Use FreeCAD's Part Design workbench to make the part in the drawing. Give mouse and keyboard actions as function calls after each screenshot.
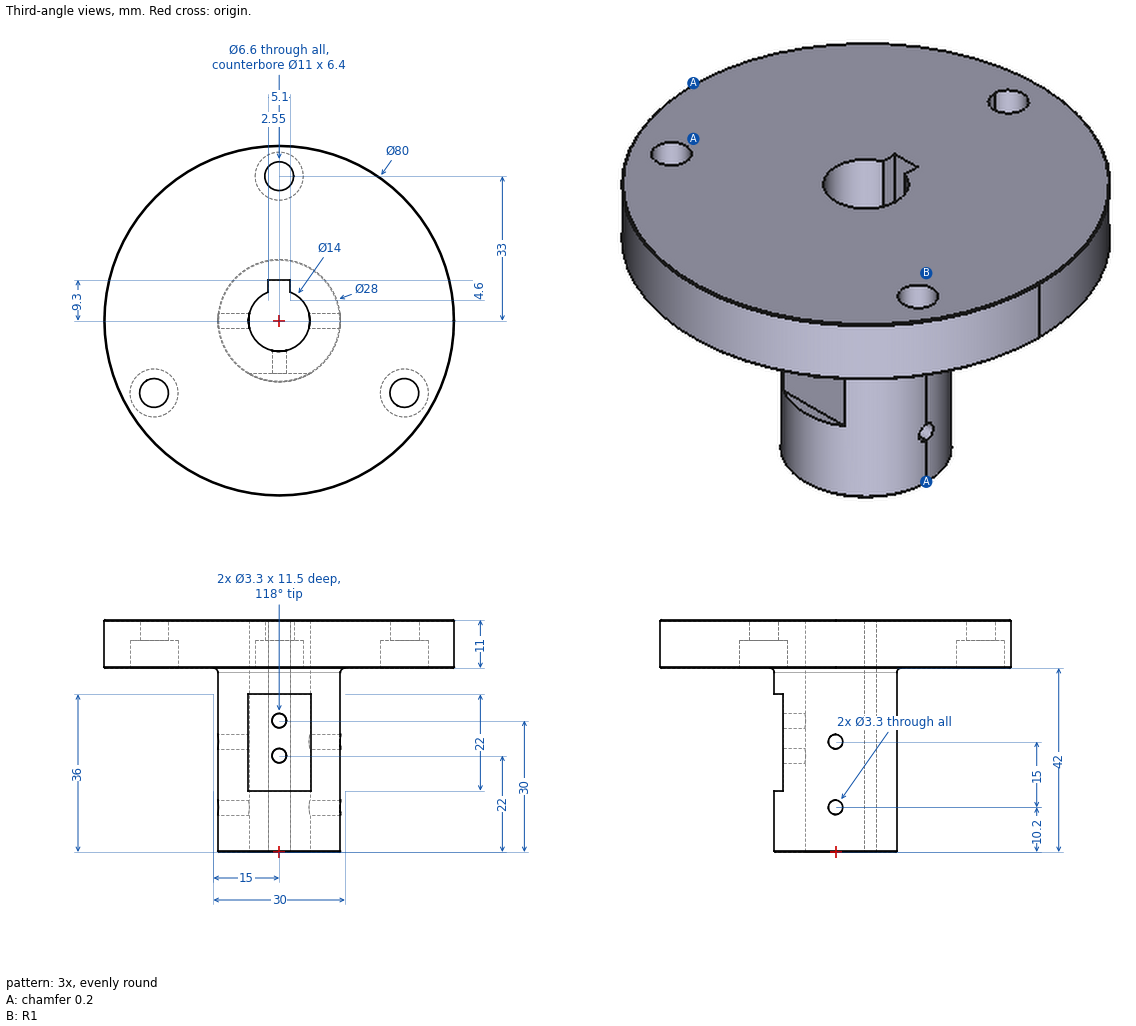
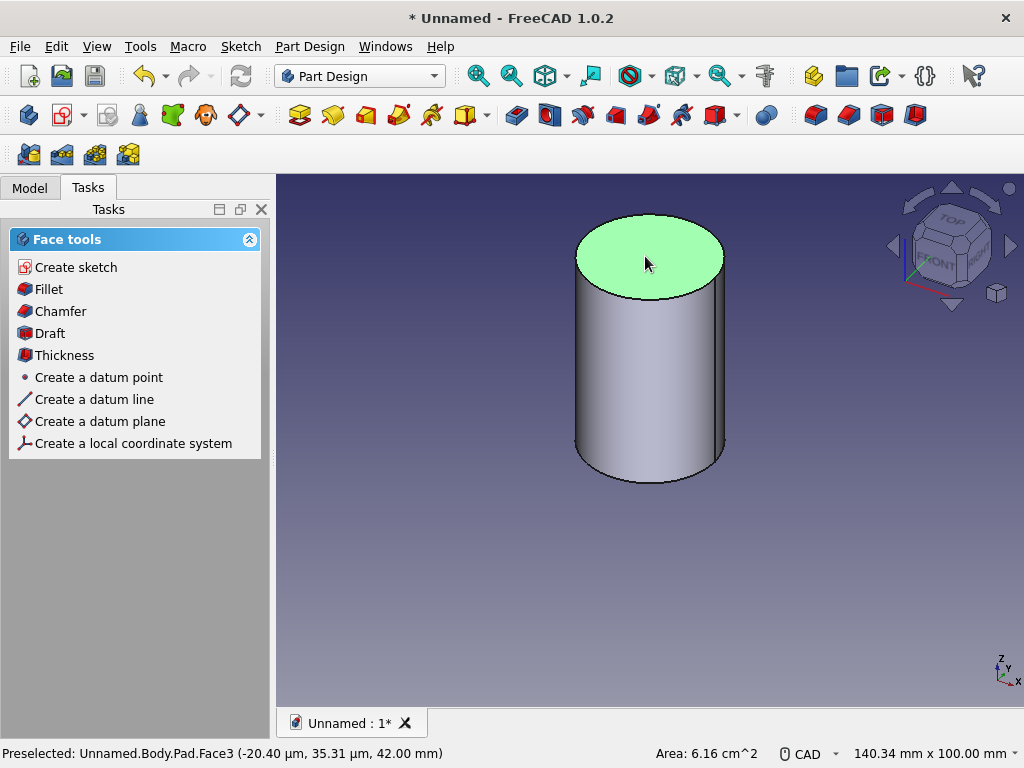
click(62, 116)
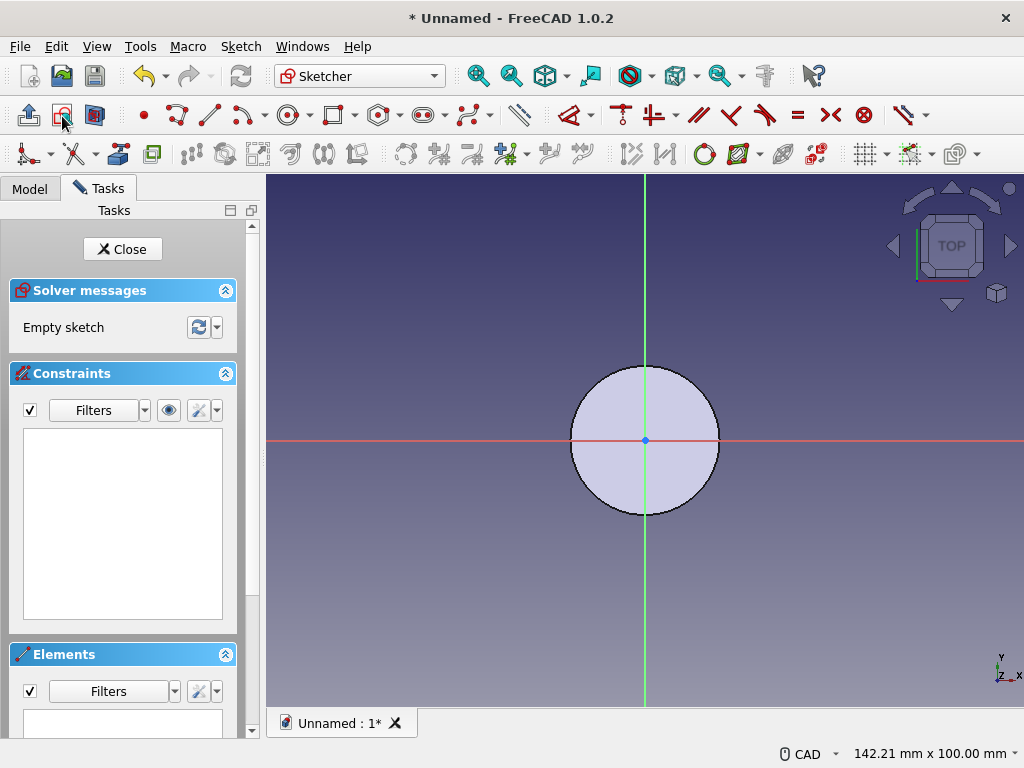
scroll(294, 440, down, 1)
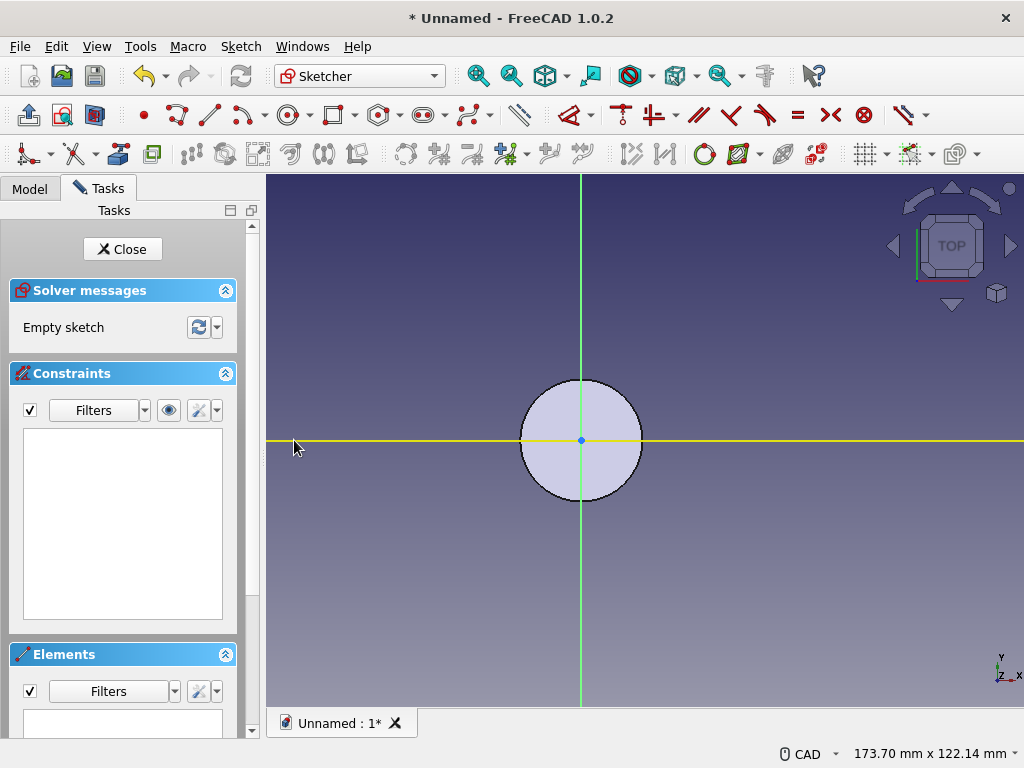
key(g)
key(c)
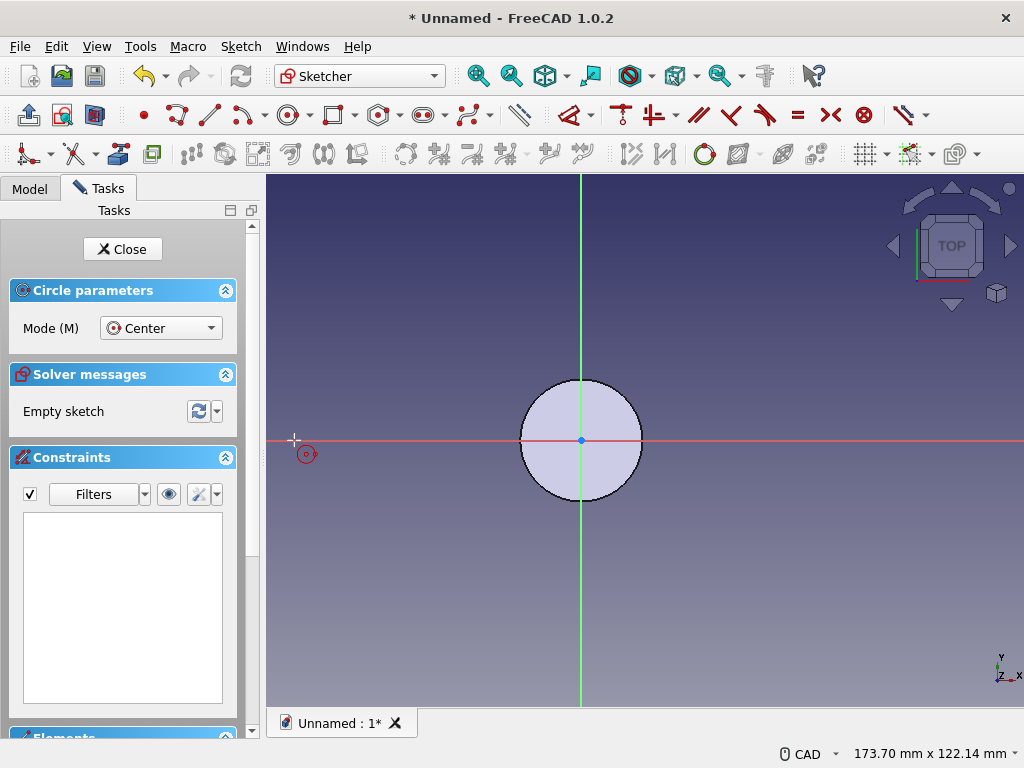
click(581, 440)
move(705, 317)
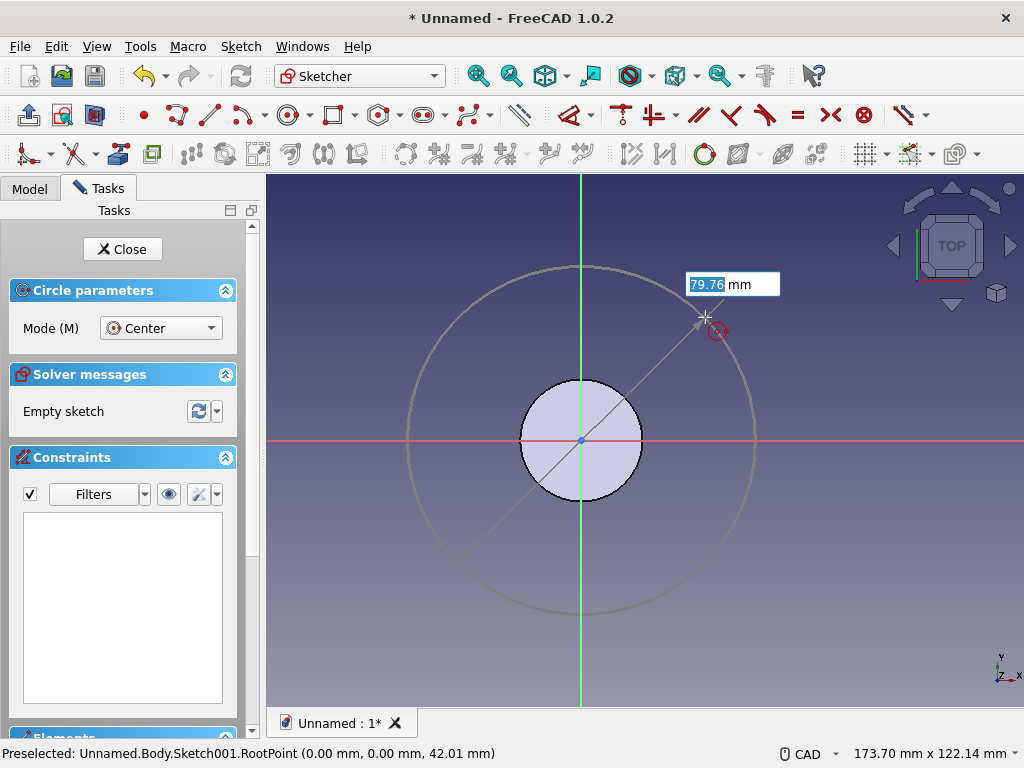
text(80)
key(Return)
key(Escape)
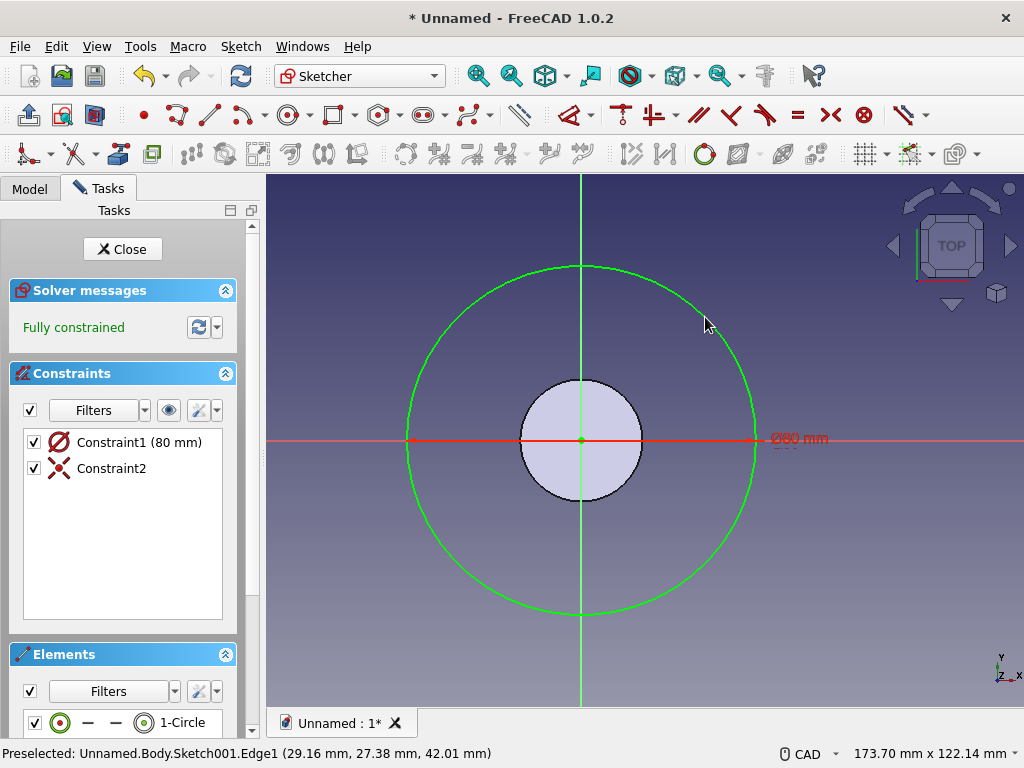
click(123, 249)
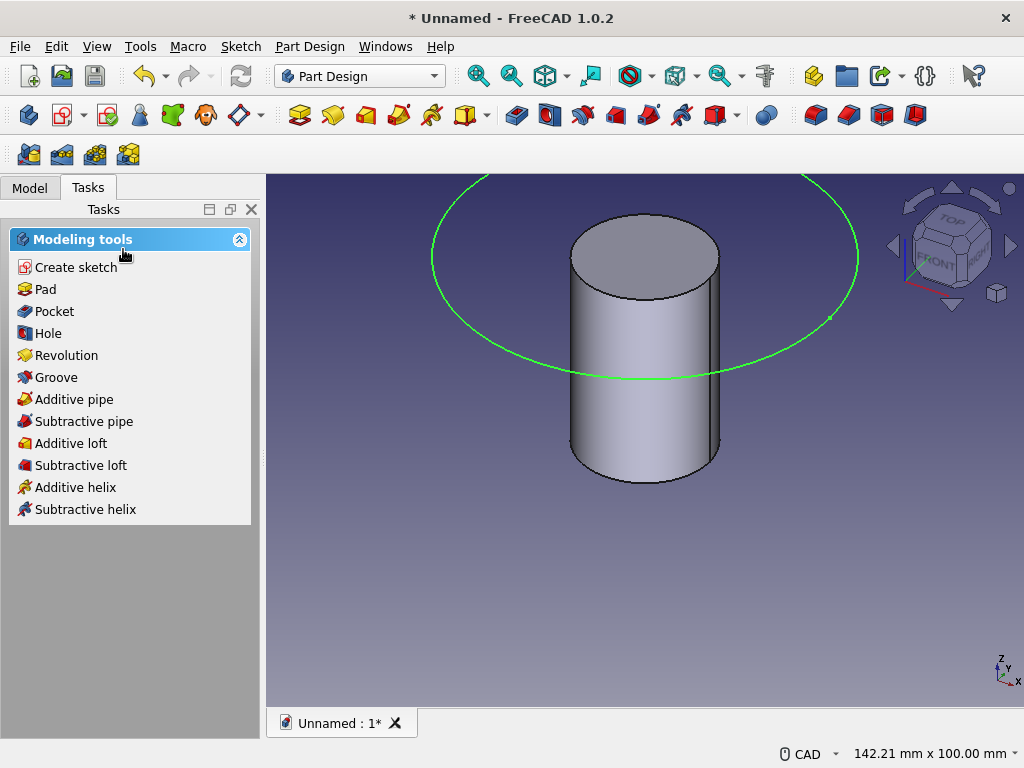
click(300, 116)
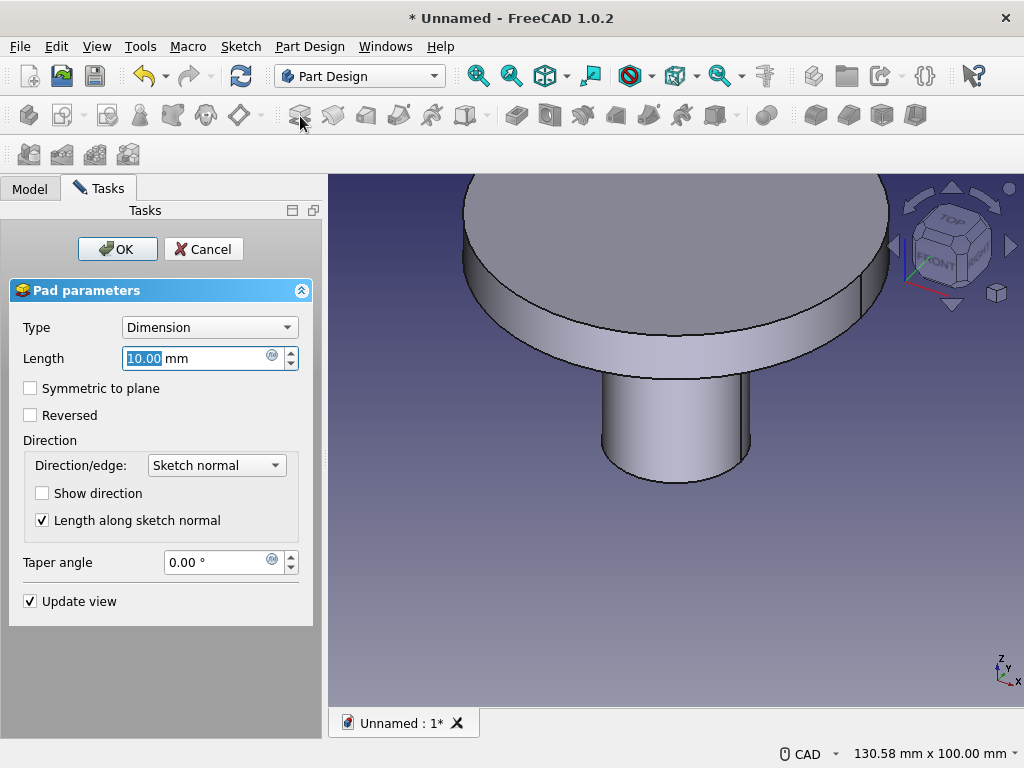
text(11)
key(Tab)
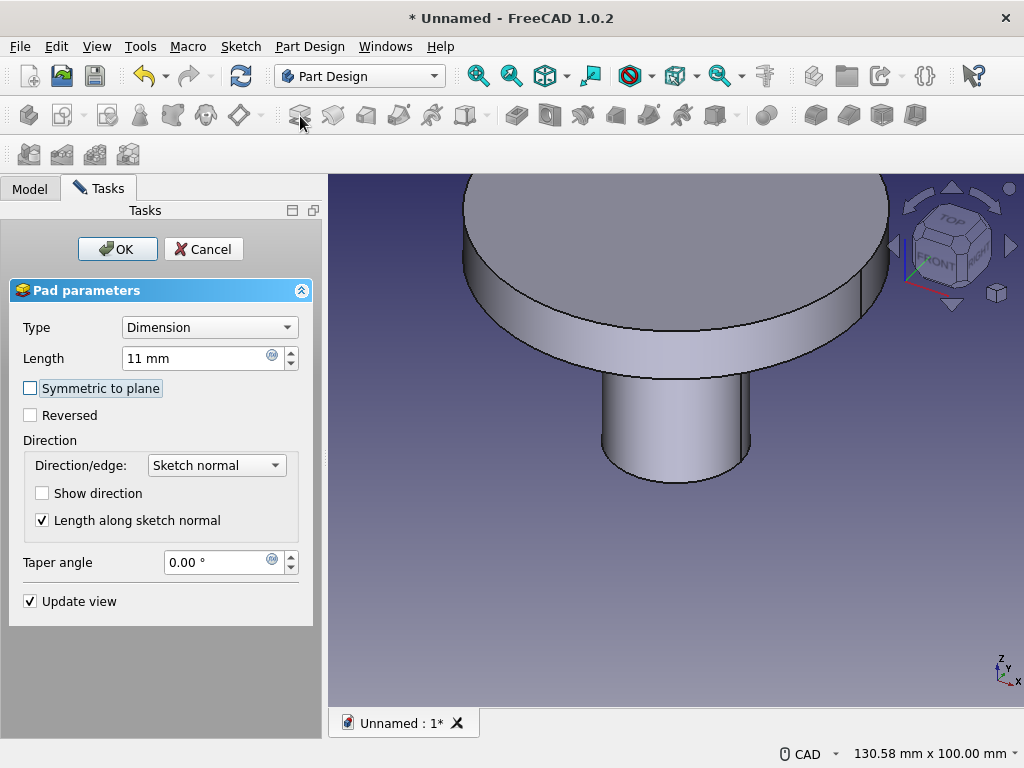
click(118, 249)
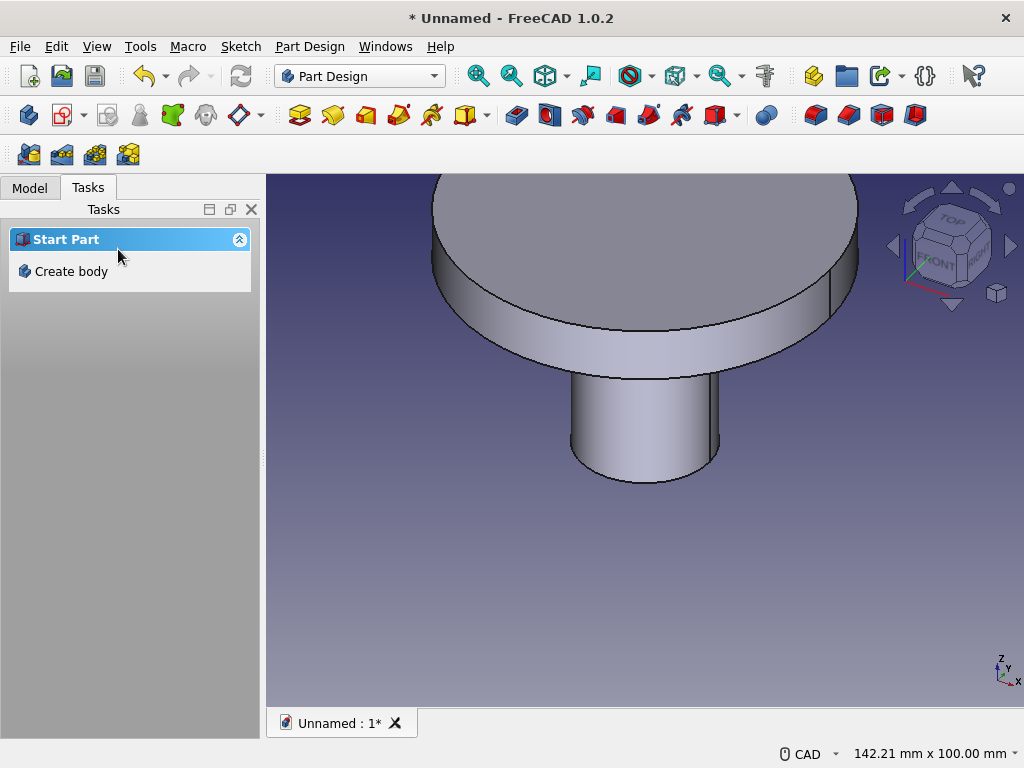
click(479, 76)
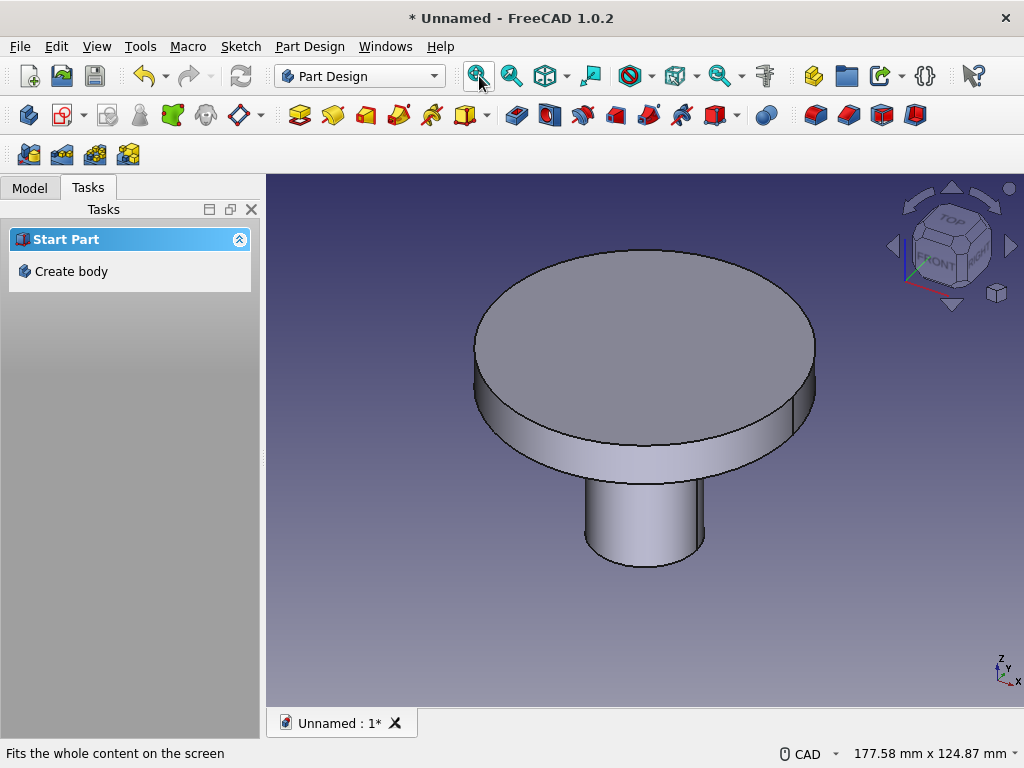
key(5)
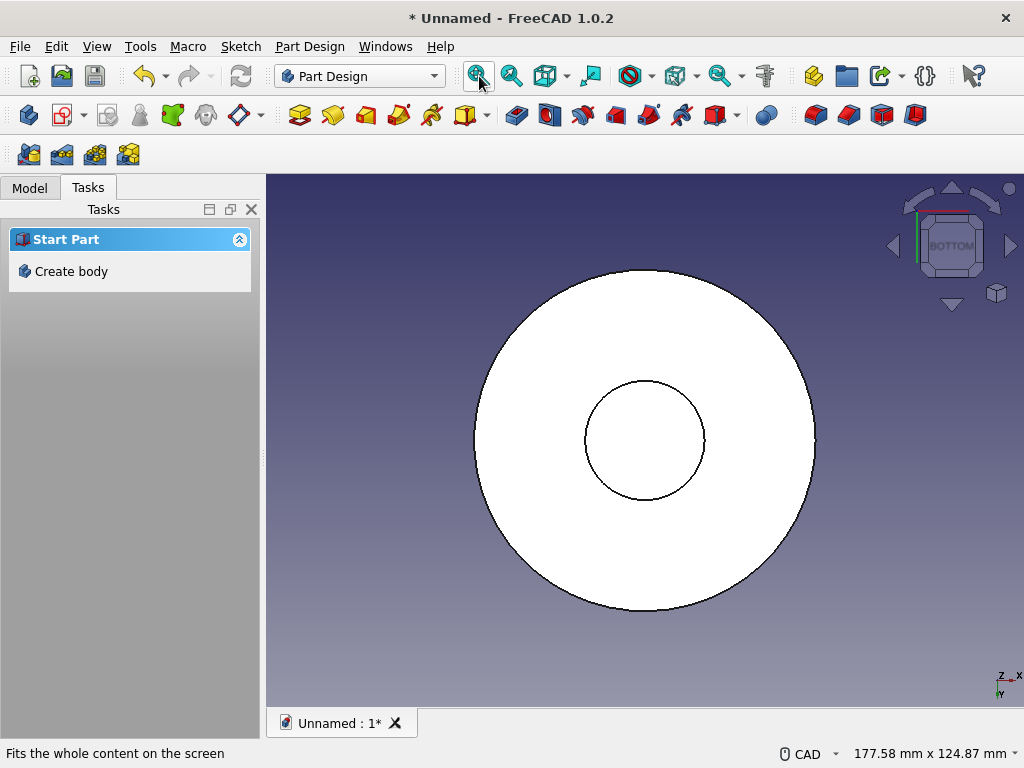
click(645, 439)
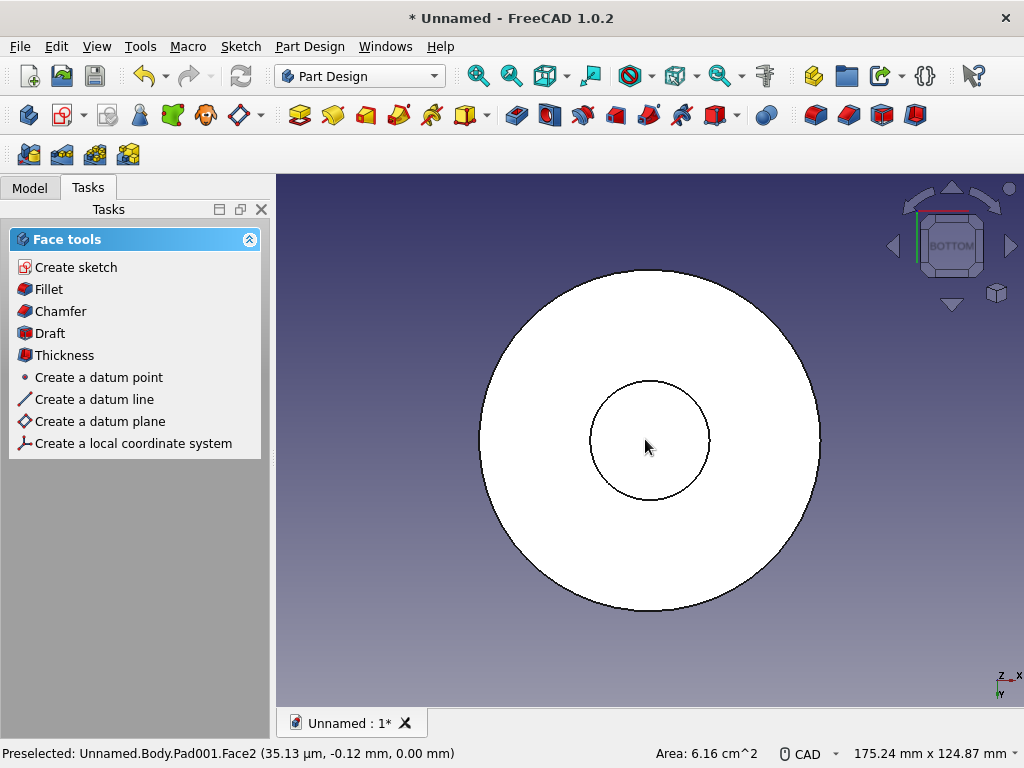
click(62, 116)